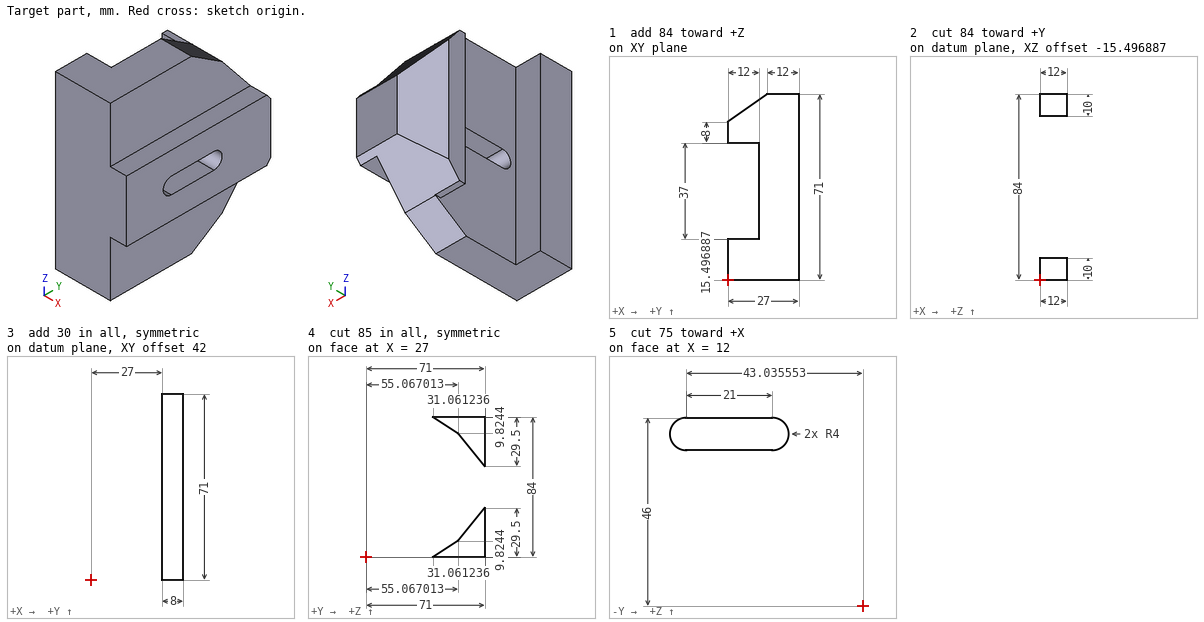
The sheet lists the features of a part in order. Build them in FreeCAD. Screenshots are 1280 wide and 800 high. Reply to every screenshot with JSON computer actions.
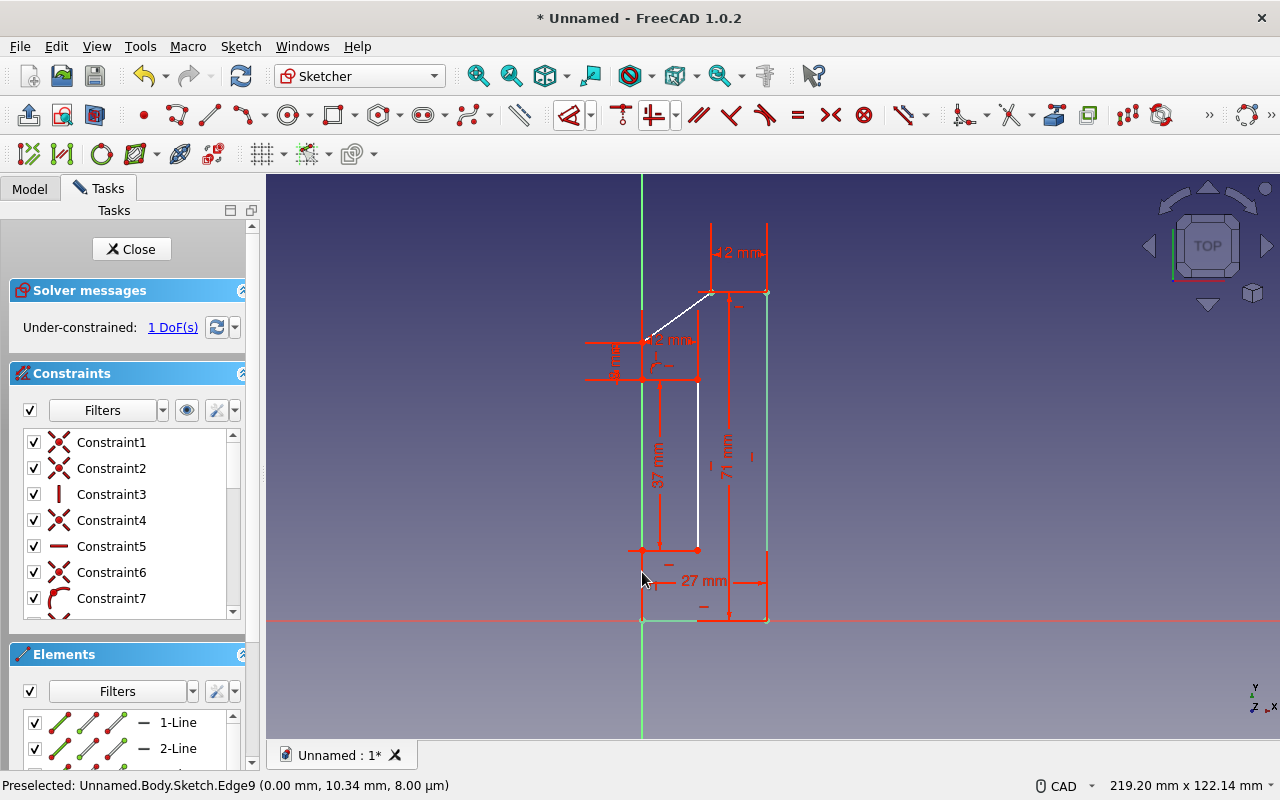
{"action": "left_click", "coordinate": [590, 116]}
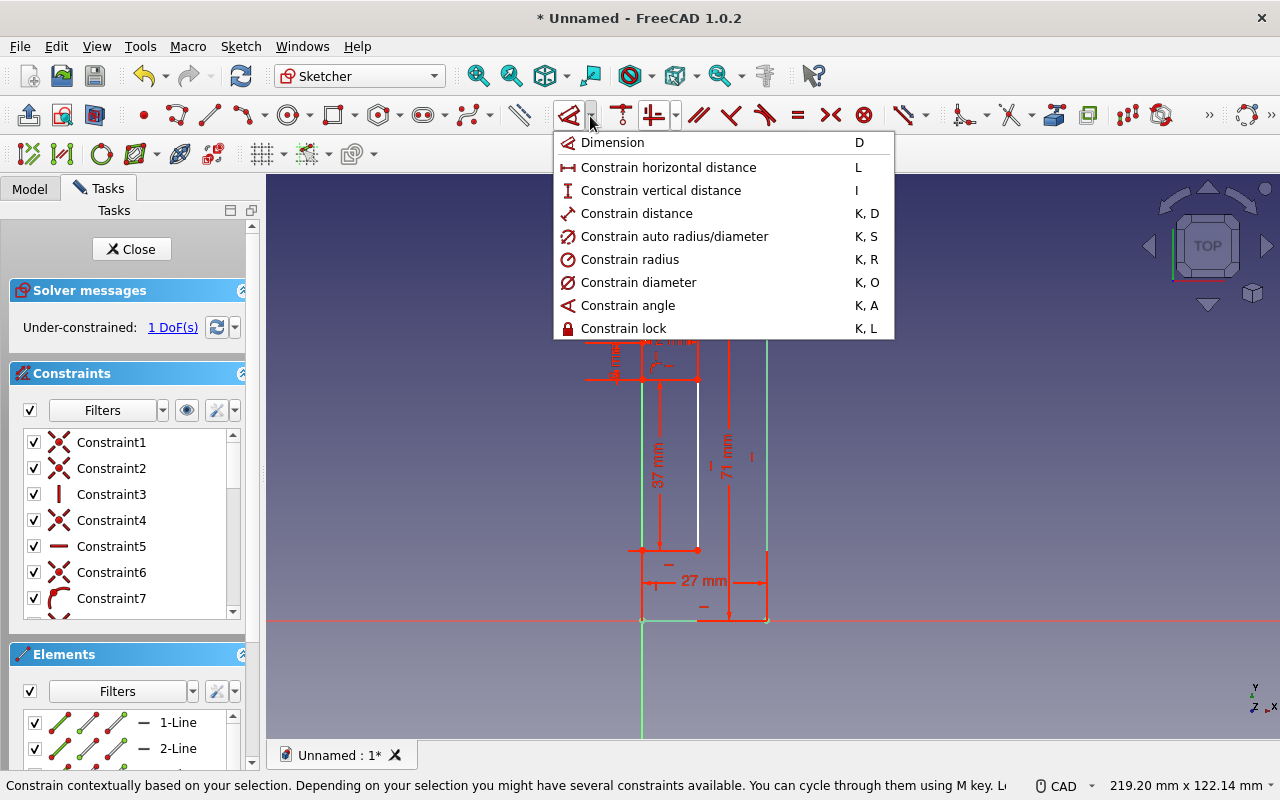
{"action": "left_click", "coordinate": [724, 190]}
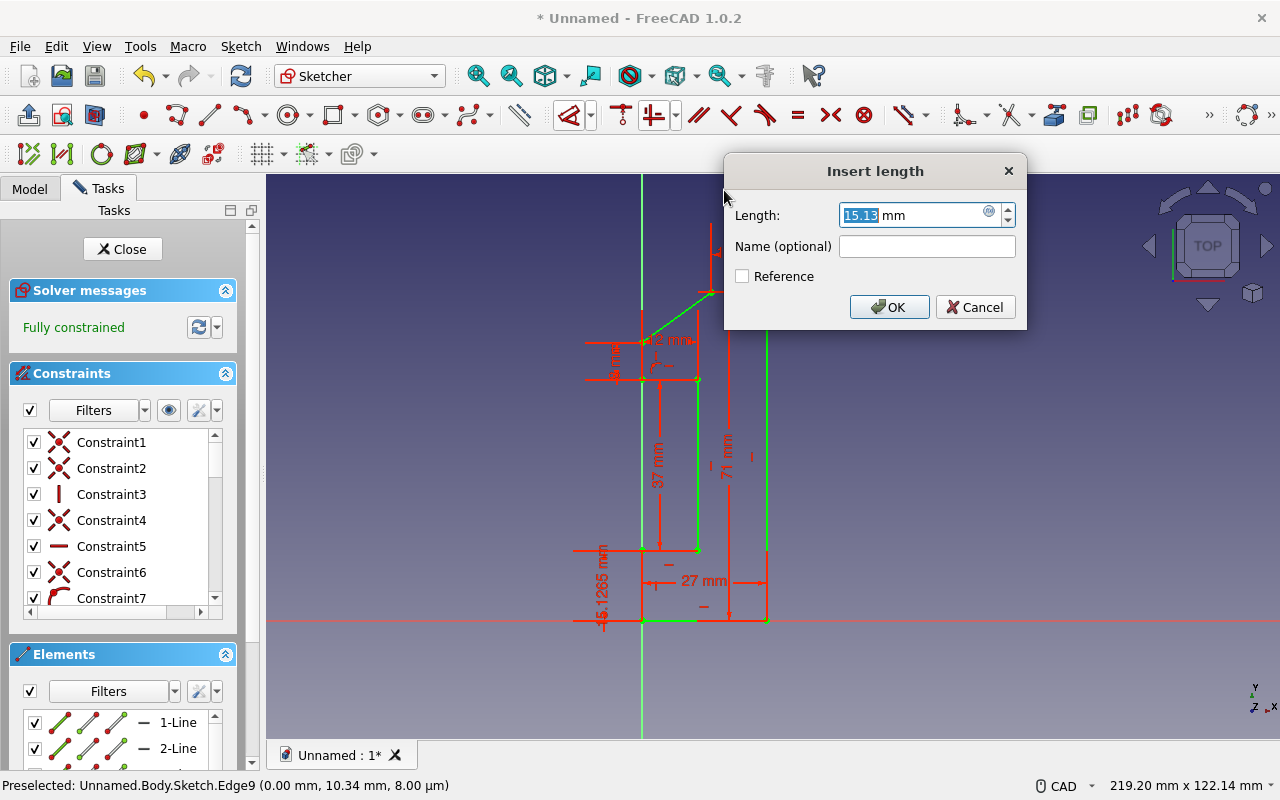
{"action": "type", "text": "15.496887"}
{"action": "key", "text": "Return"}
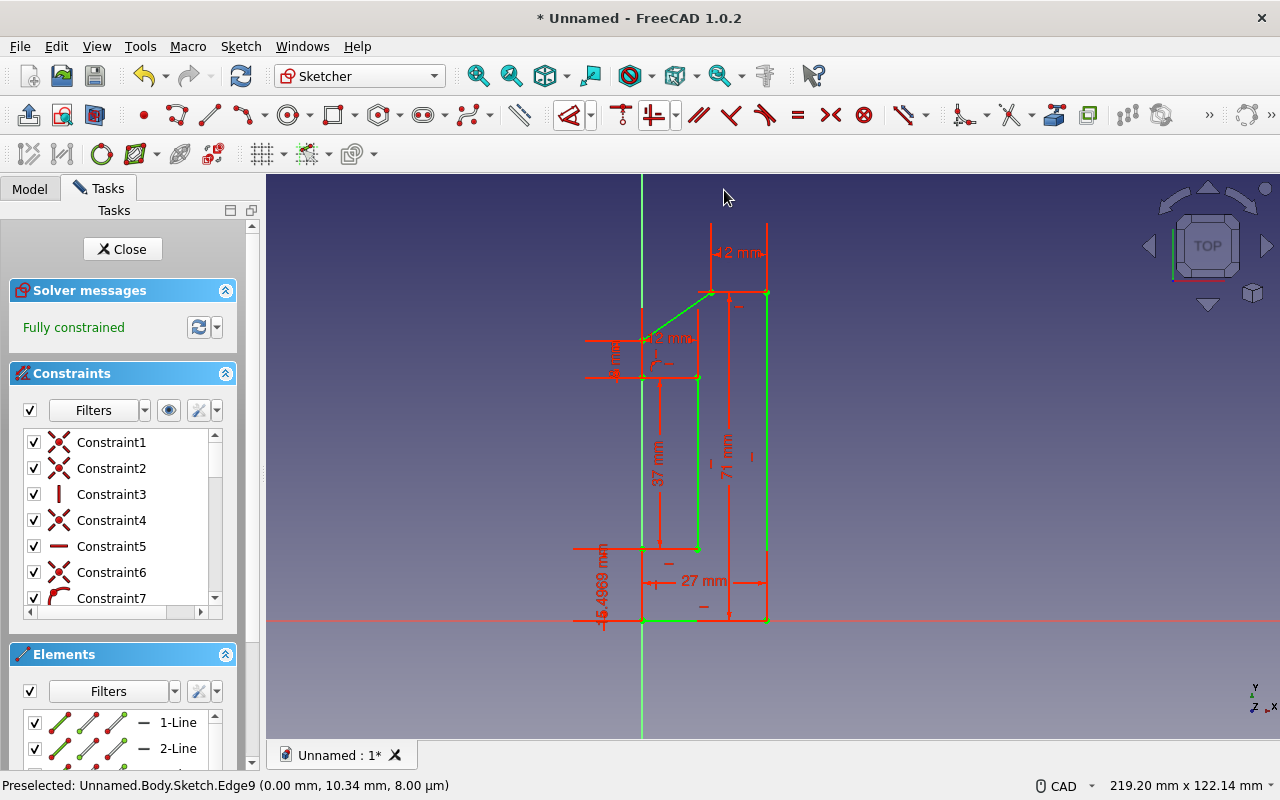
{"action": "left_click", "coordinate": [123, 249]}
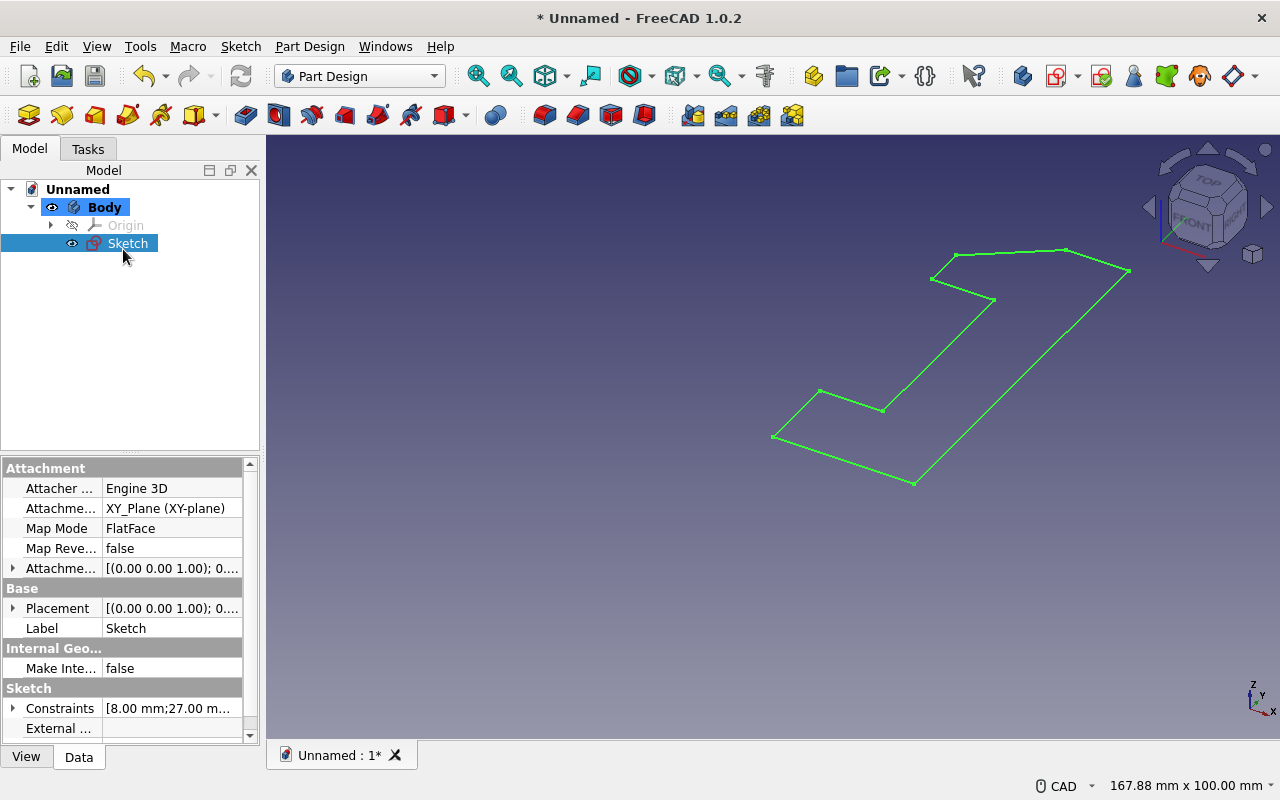
{"action": "left_click", "coordinate": [29, 116]}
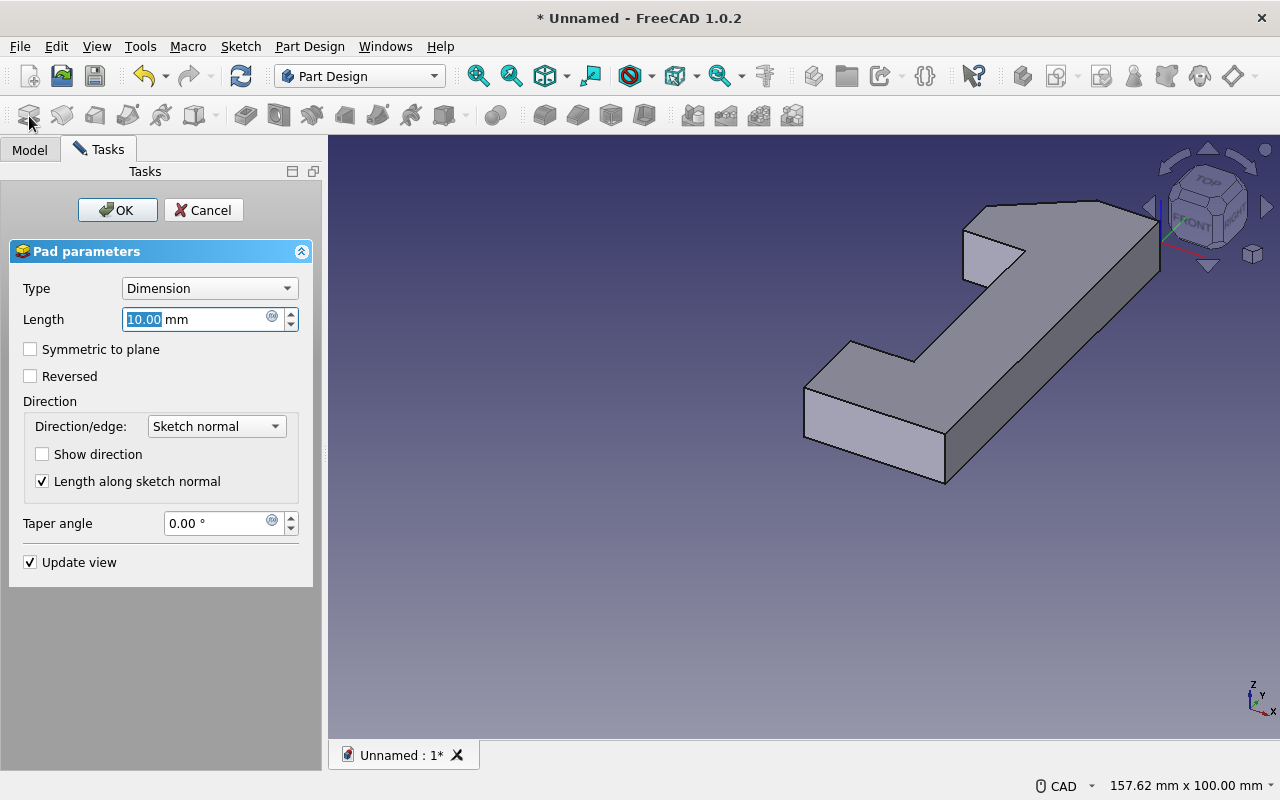
{"action": "type", "text": "84"}
{"action": "key", "text": "Tab"}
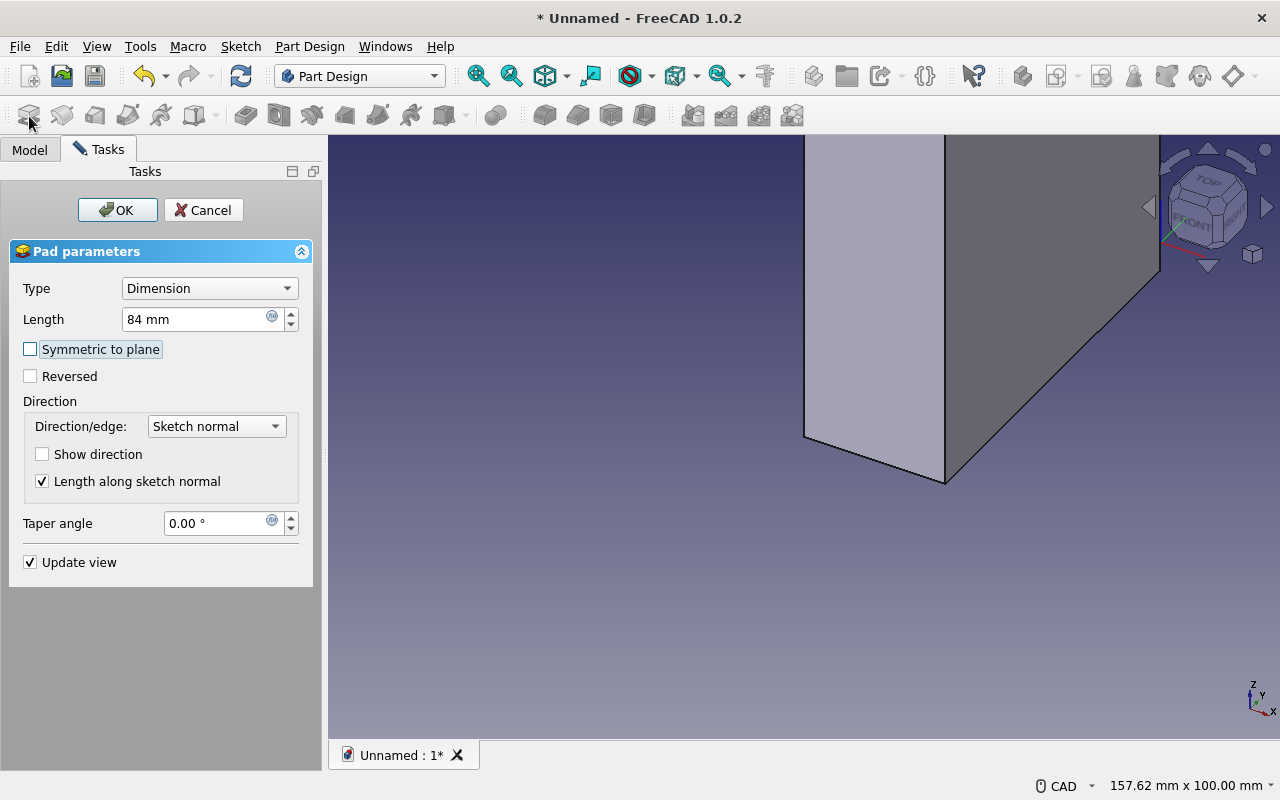
{"action": "left_click", "coordinate": [118, 210]}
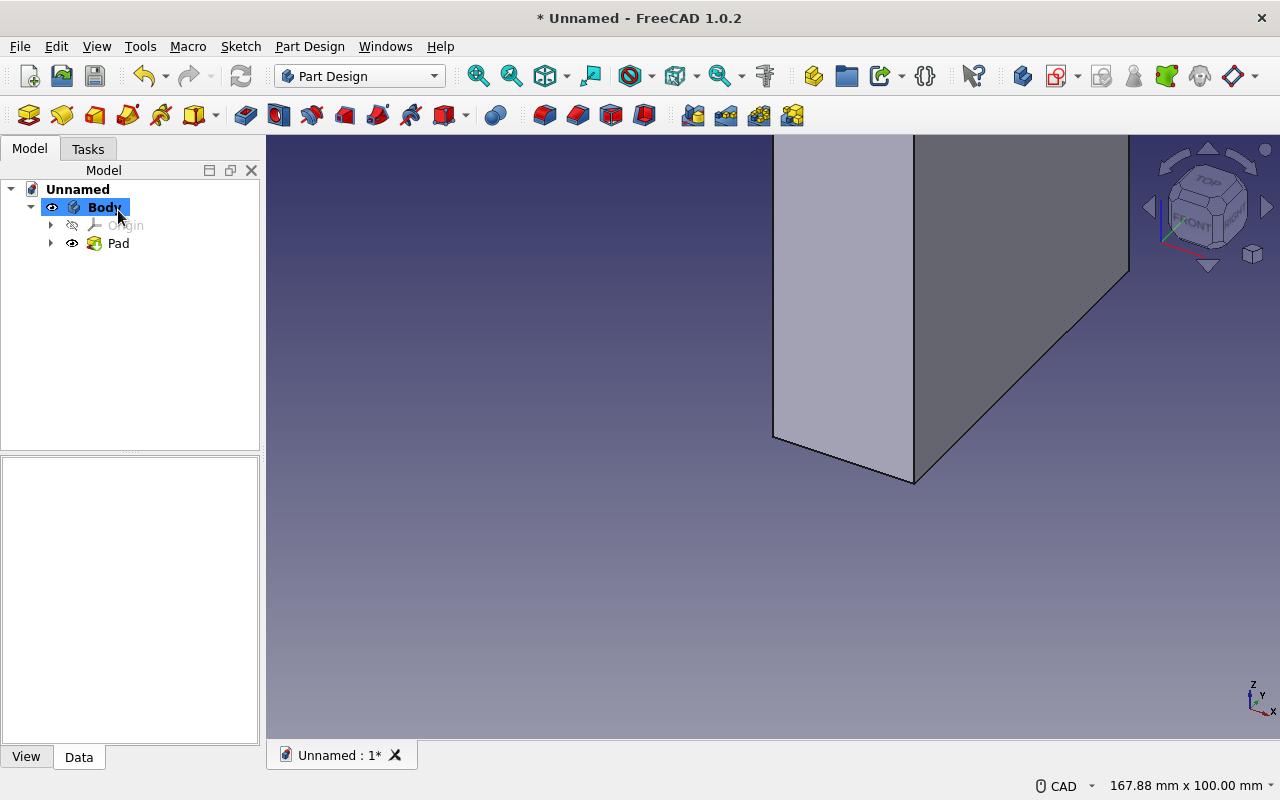
{"action": "left_click", "coordinate": [479, 76]}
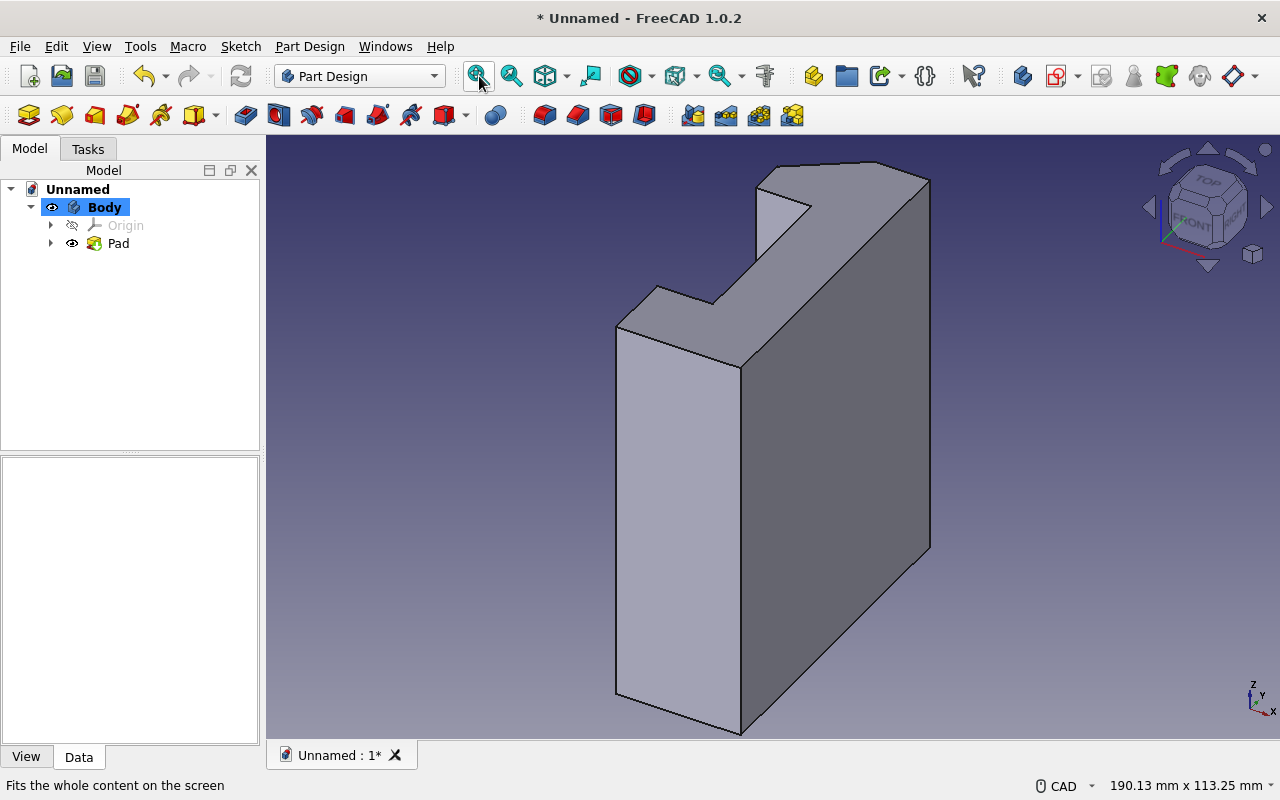
{"action": "left_click", "coordinate": [51, 225]}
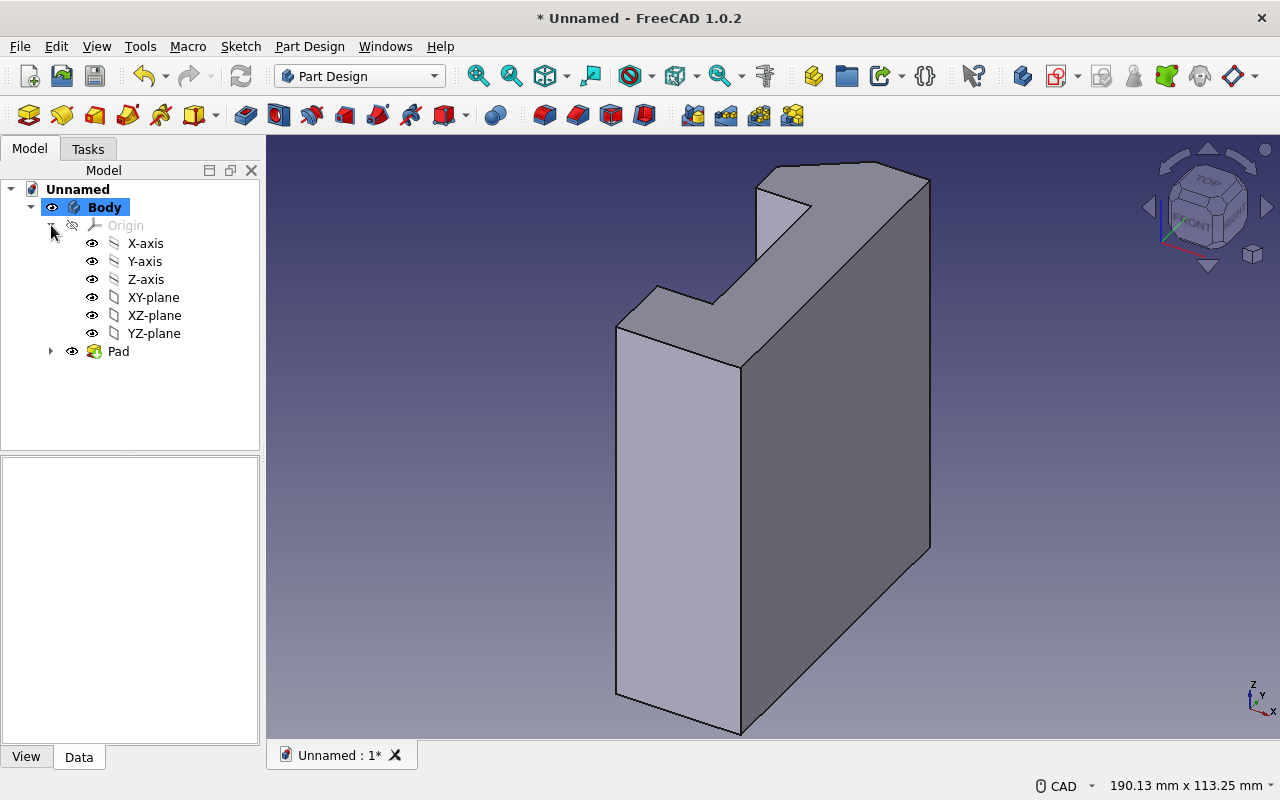
{"action": "left_click", "coordinate": [137, 315]}